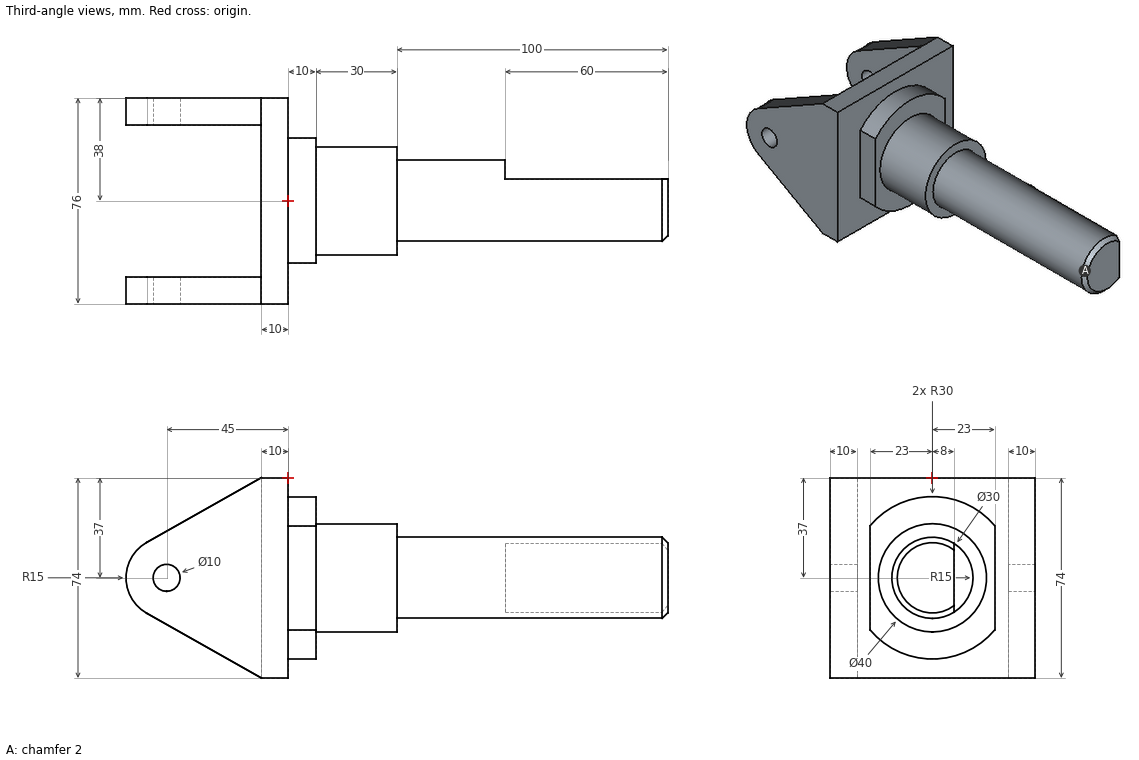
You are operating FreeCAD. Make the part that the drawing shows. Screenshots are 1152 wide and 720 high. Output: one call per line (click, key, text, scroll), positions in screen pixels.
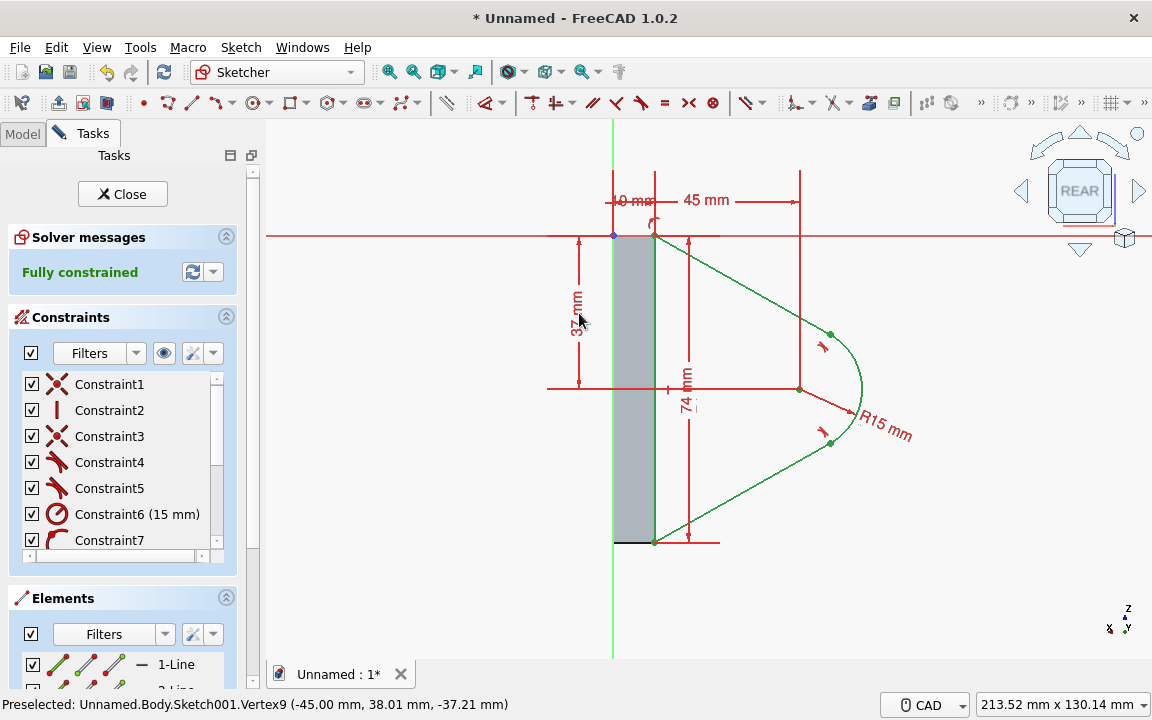
click(123, 194)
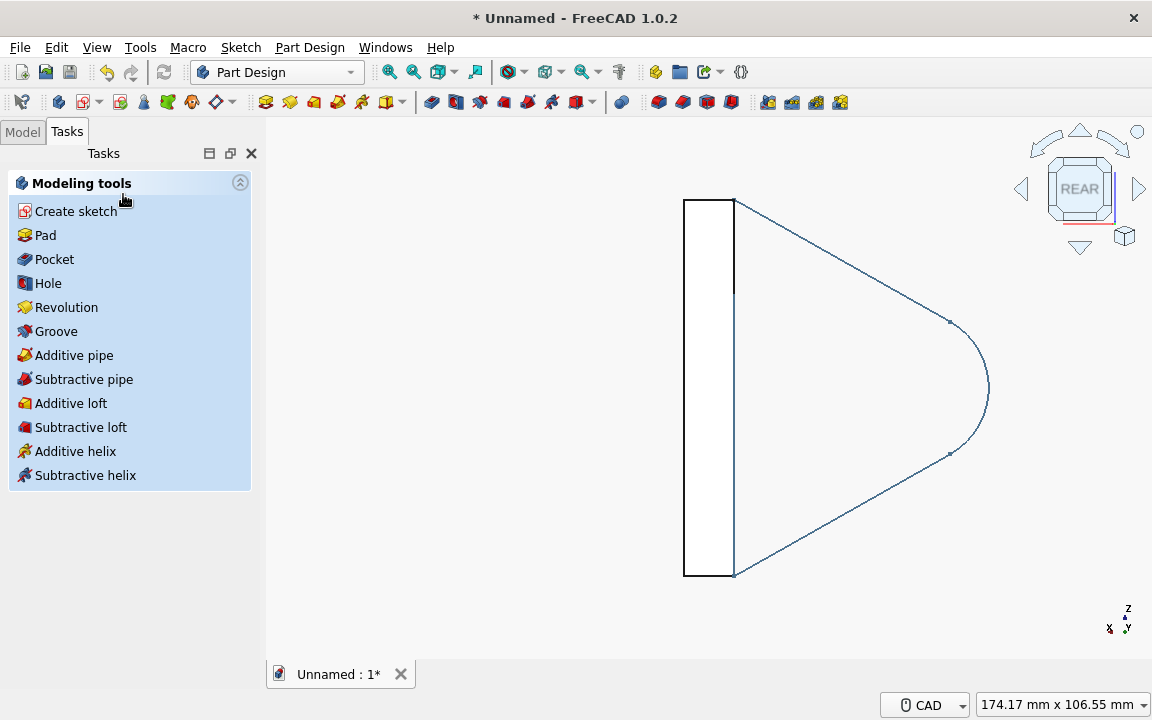
click(266, 102)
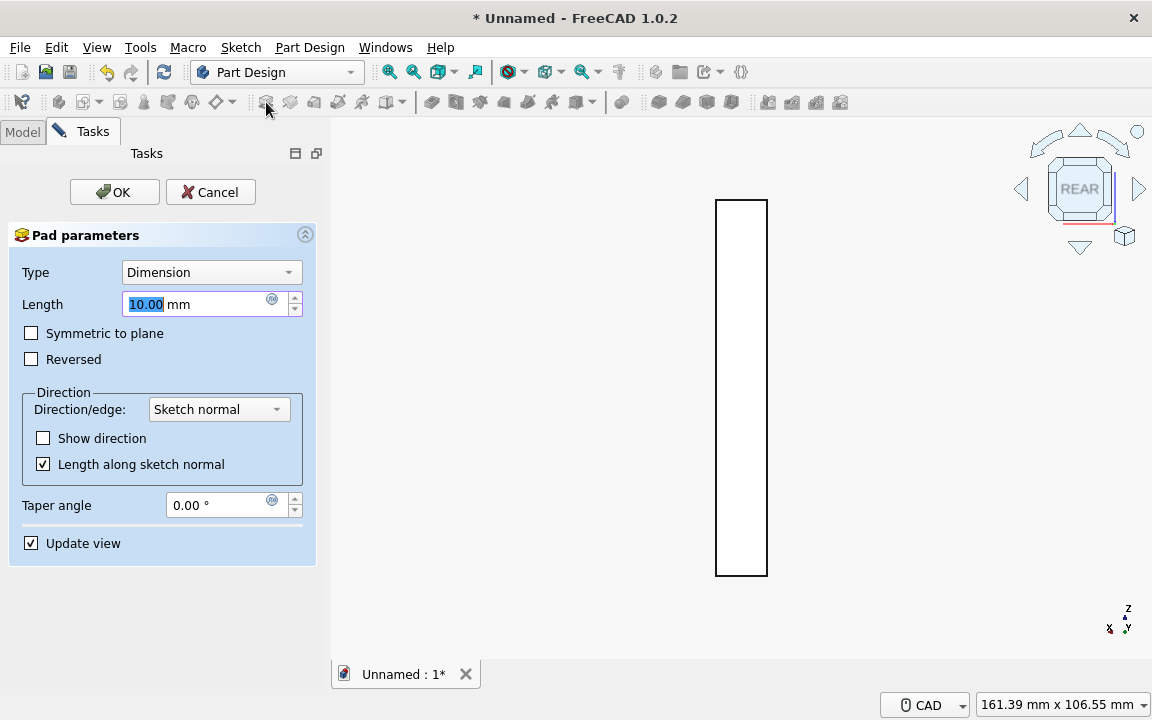
text(10)
key(Tab)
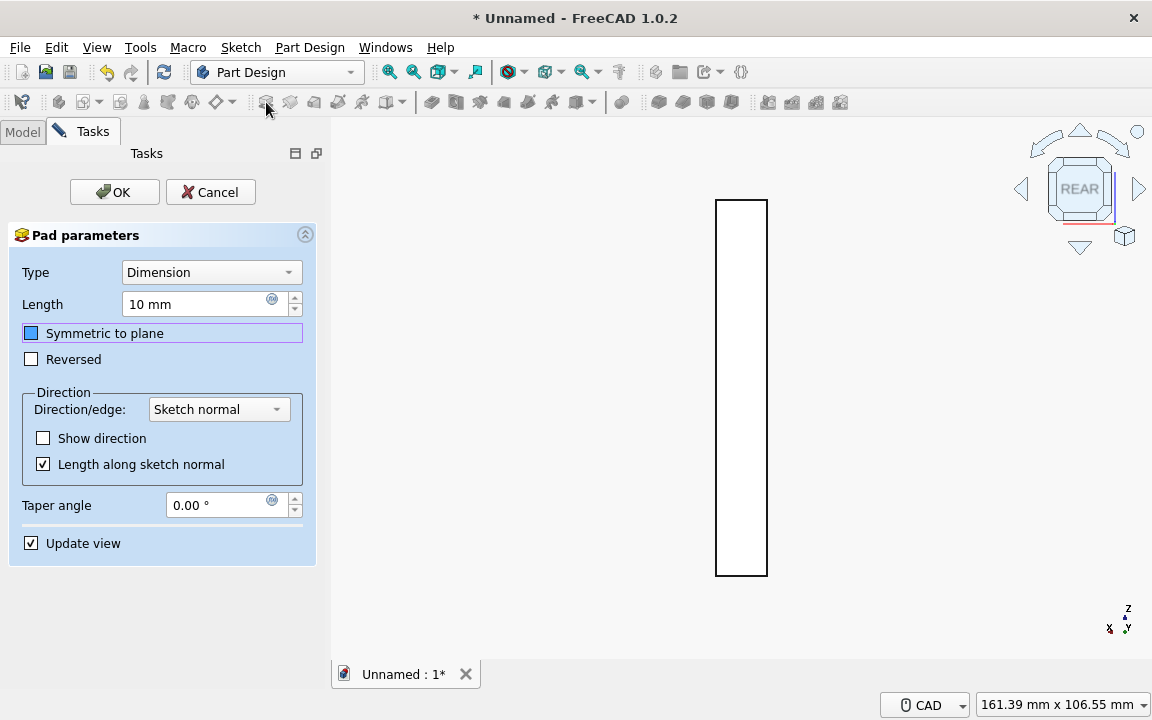
click(30, 359)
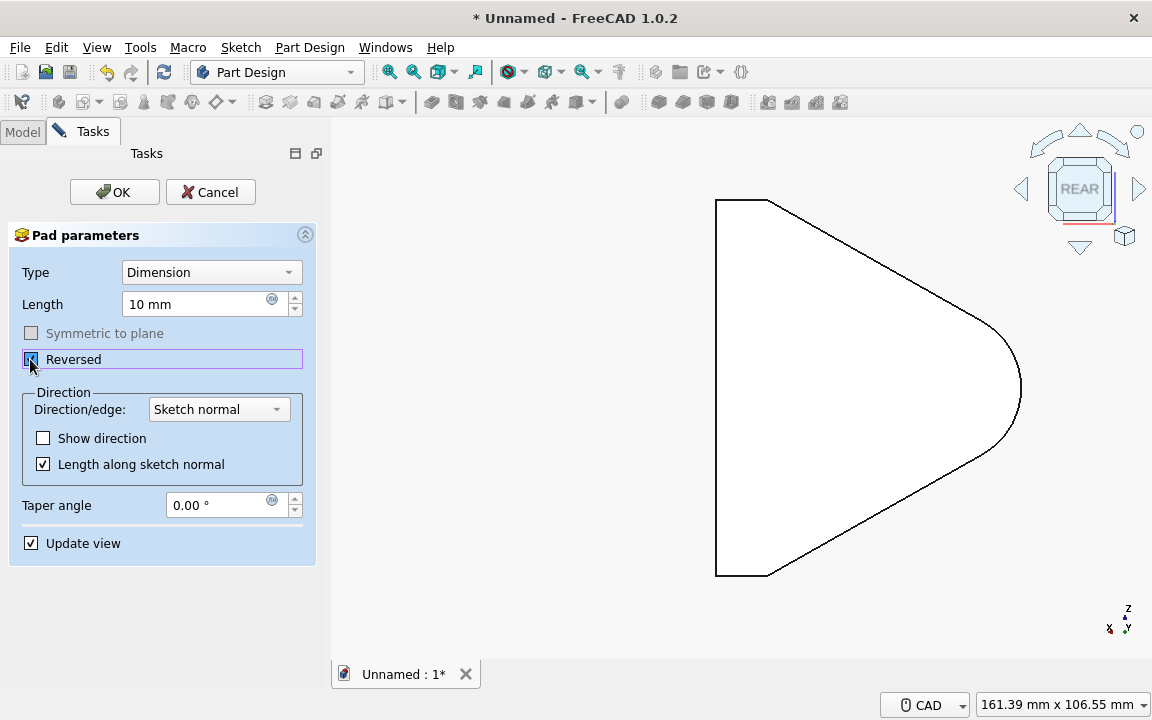
click(115, 192)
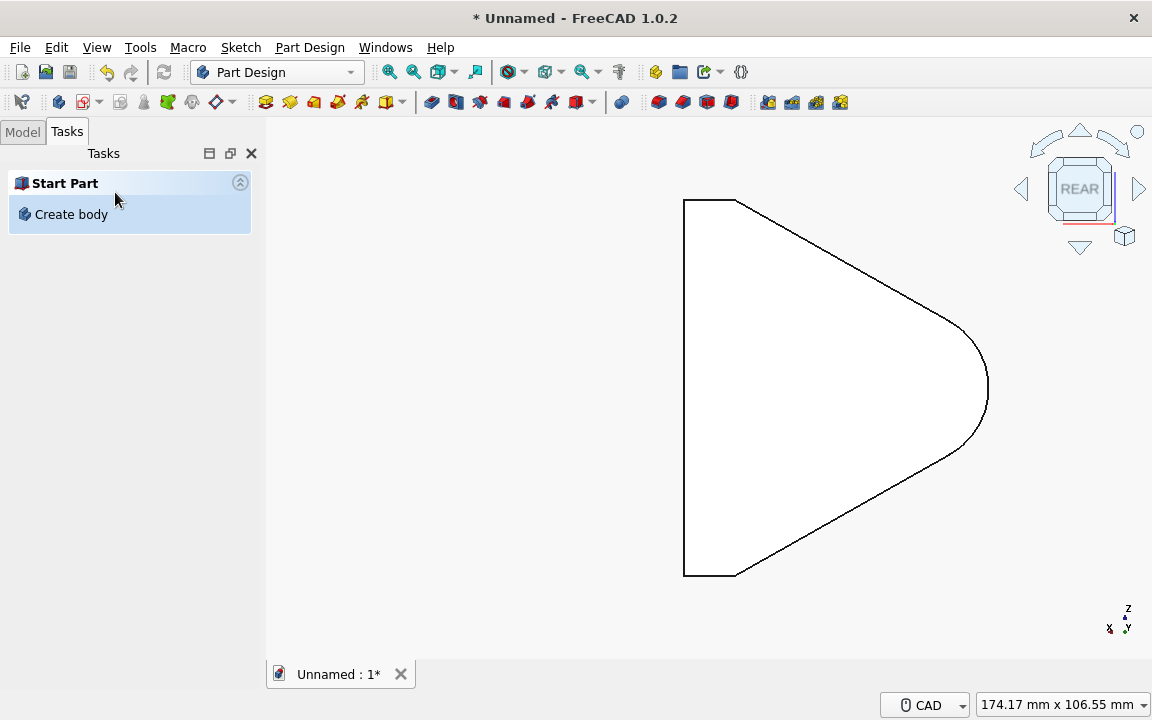
click(23, 131)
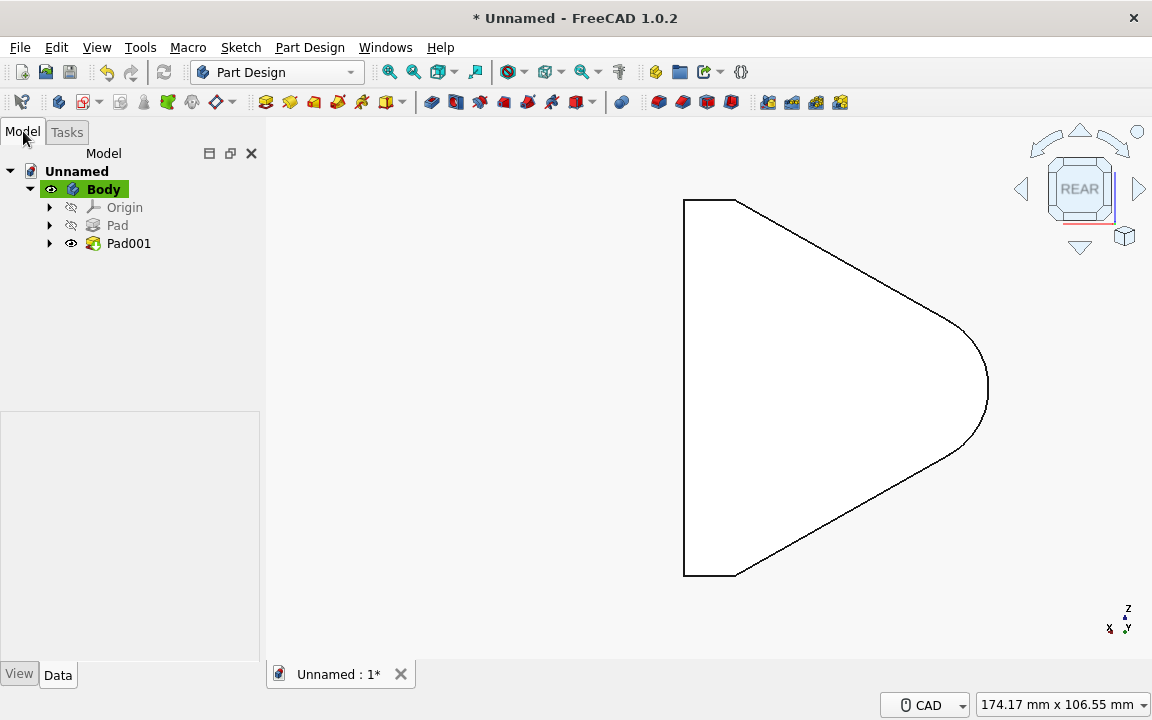
click(50, 207)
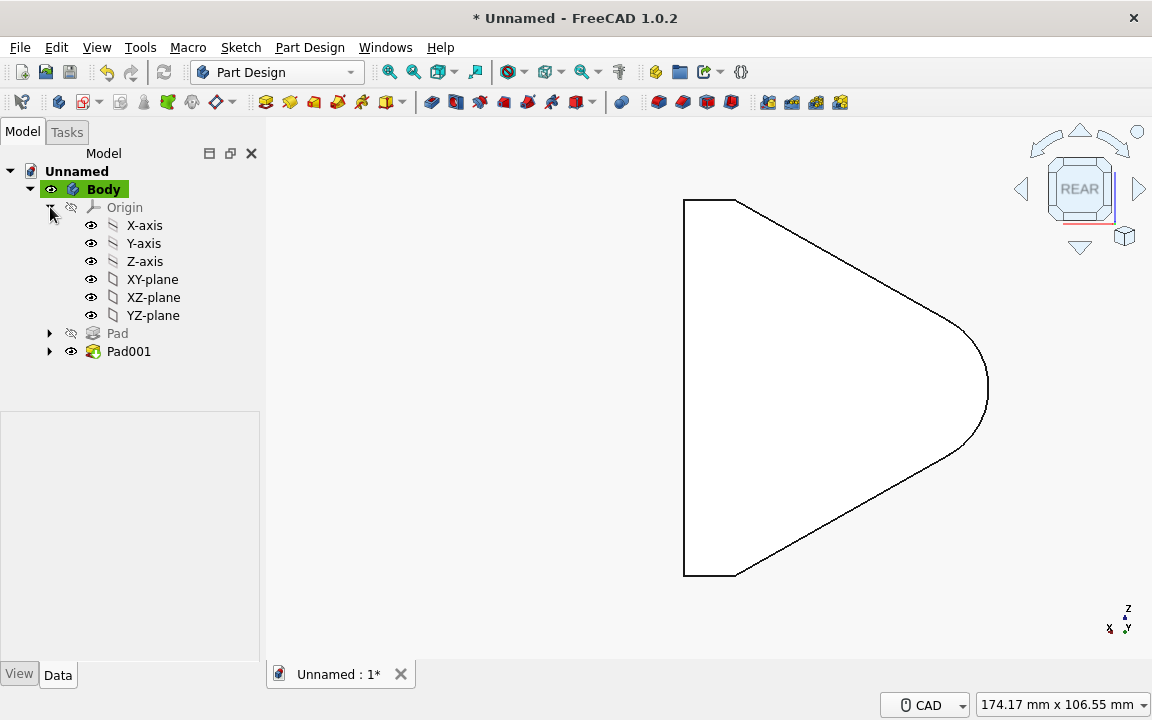
click(136, 297)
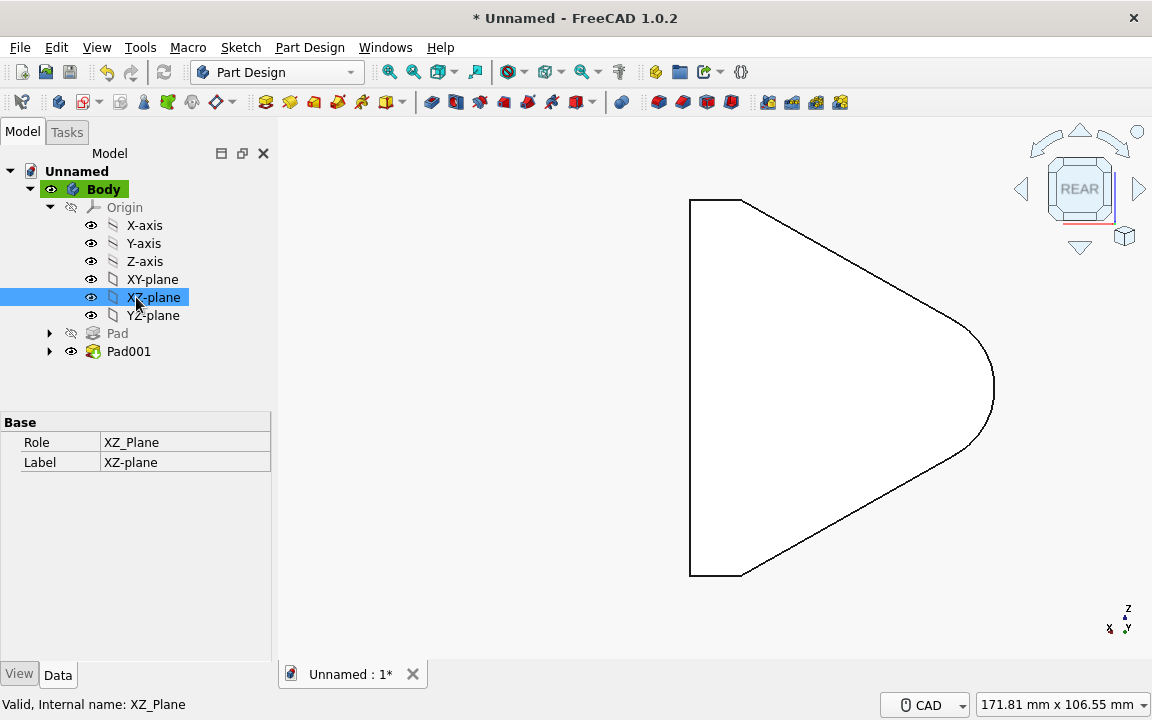
click(216, 102)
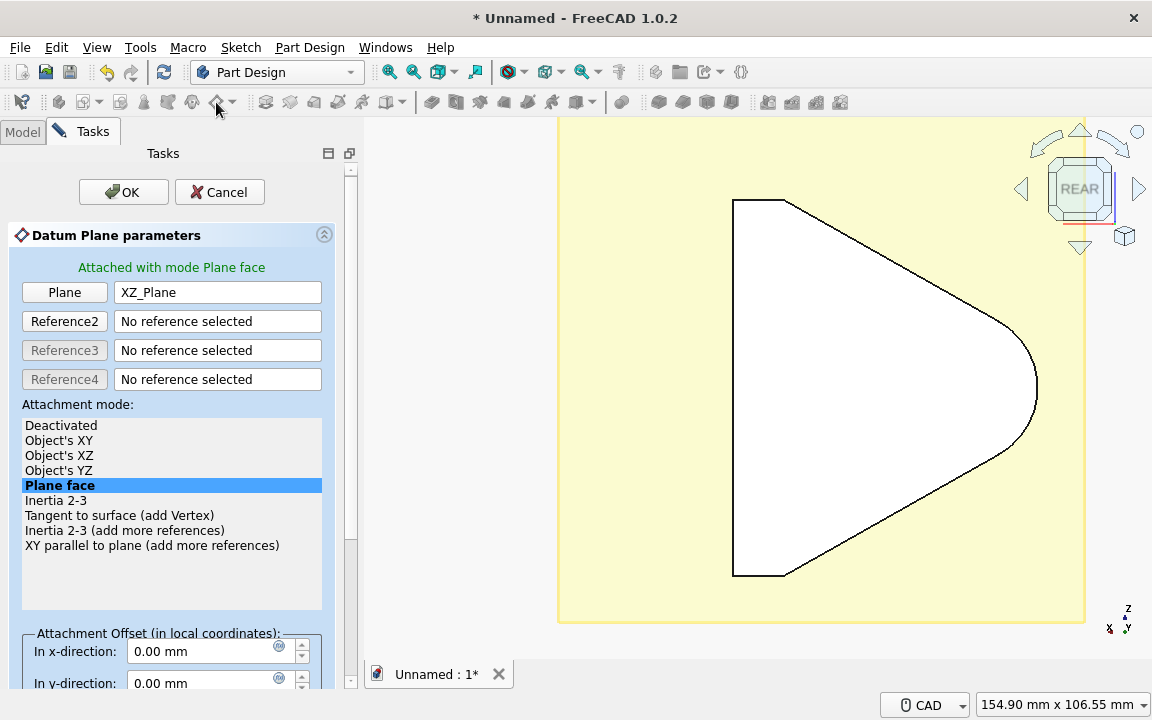
scroll(351, 426, down, 2)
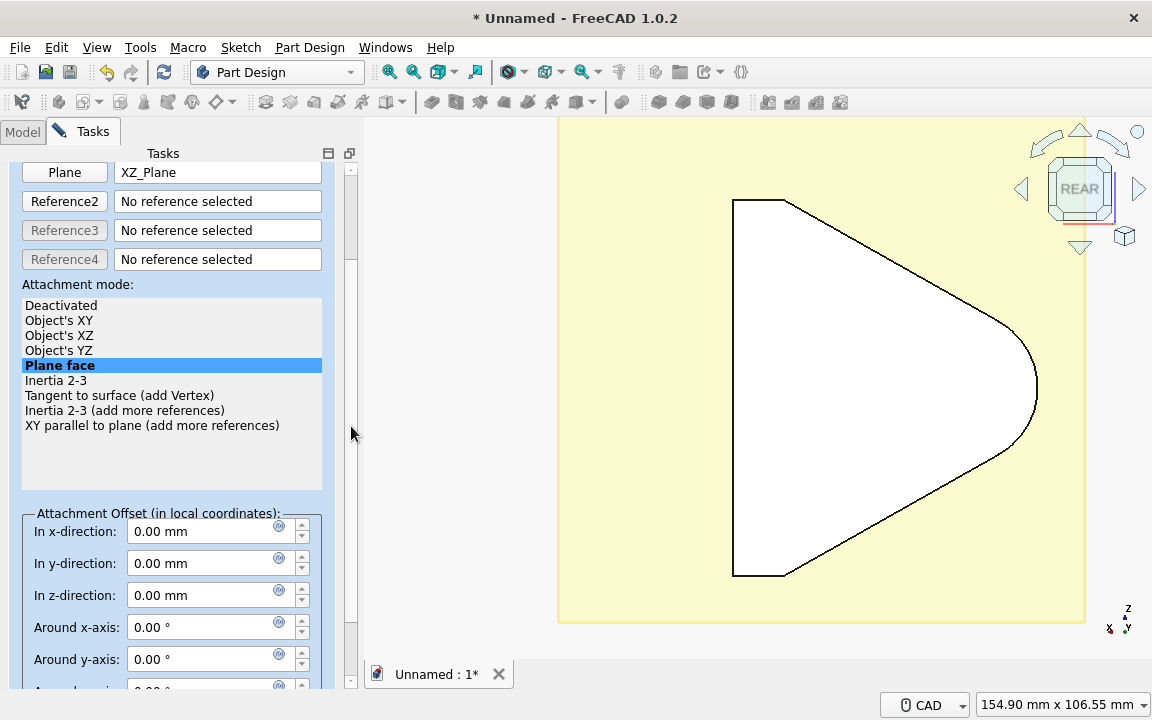
triple_click(210, 595)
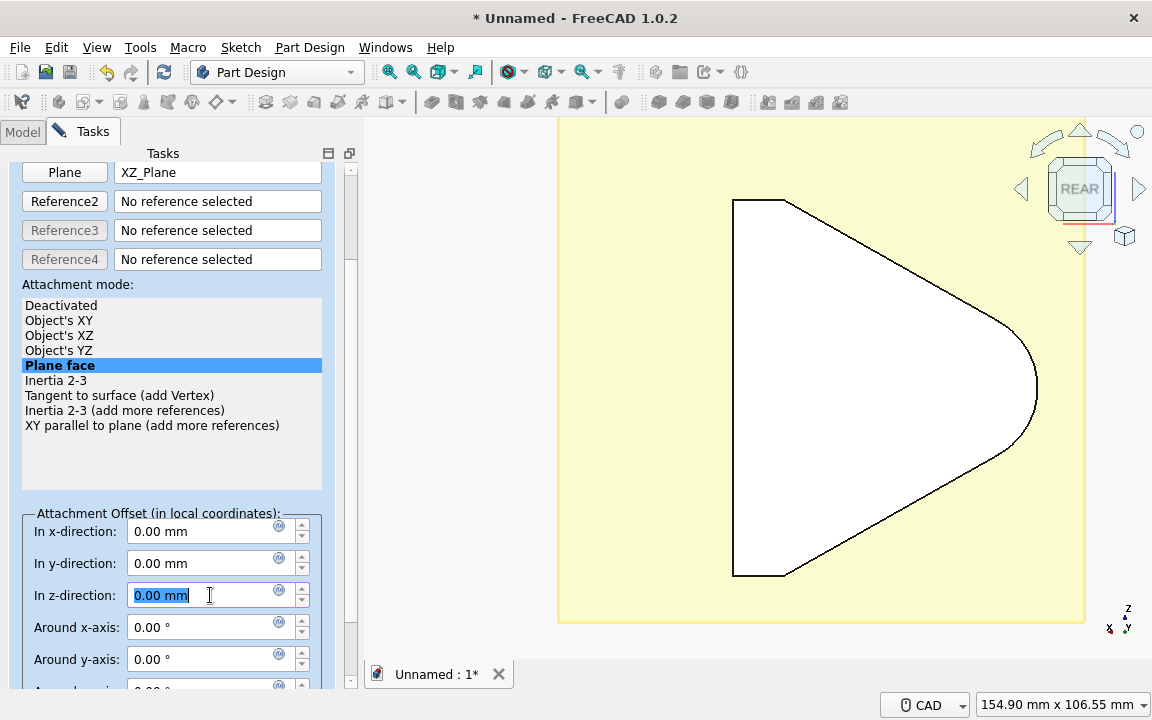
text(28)
key(Tab)